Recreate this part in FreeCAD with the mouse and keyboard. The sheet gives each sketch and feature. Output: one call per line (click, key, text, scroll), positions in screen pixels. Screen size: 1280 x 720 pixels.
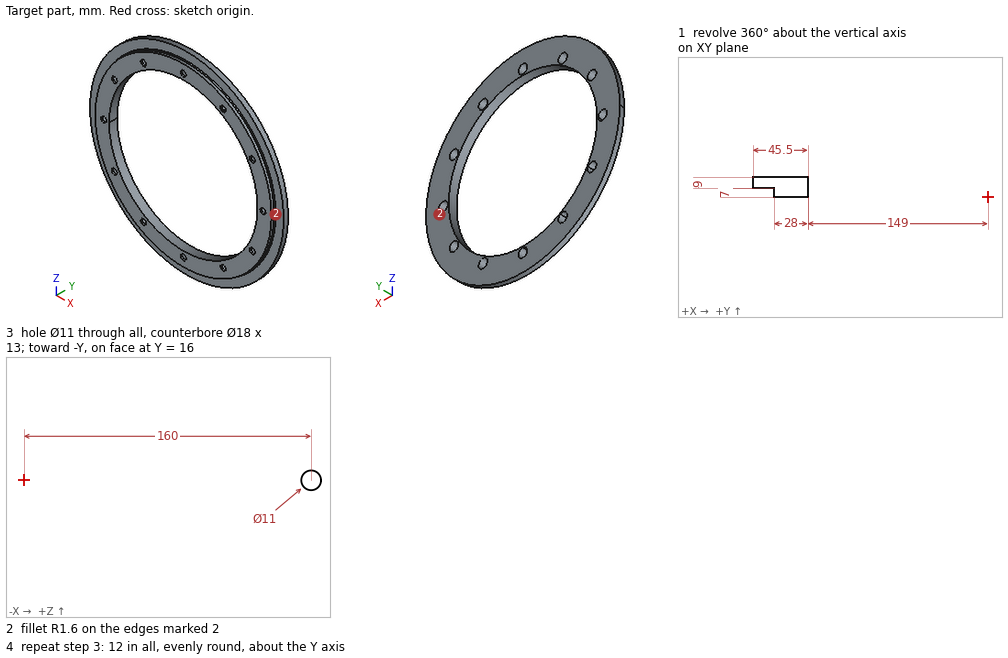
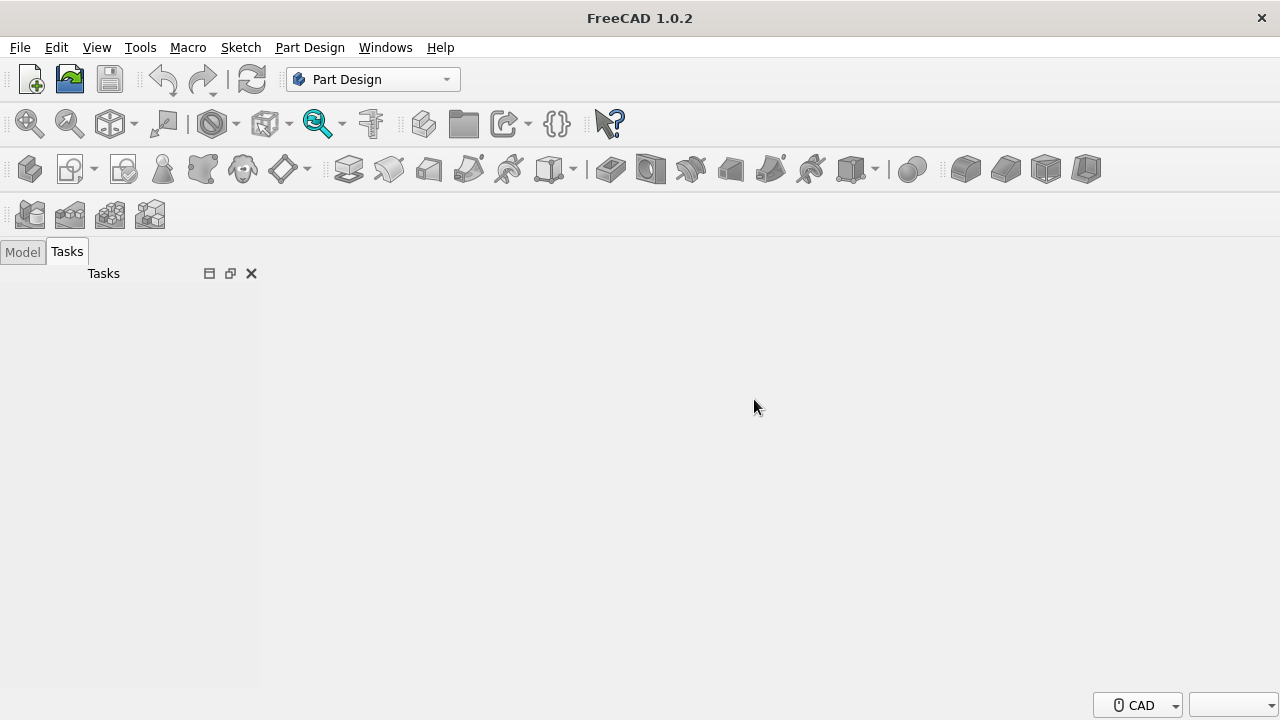
click(30, 80)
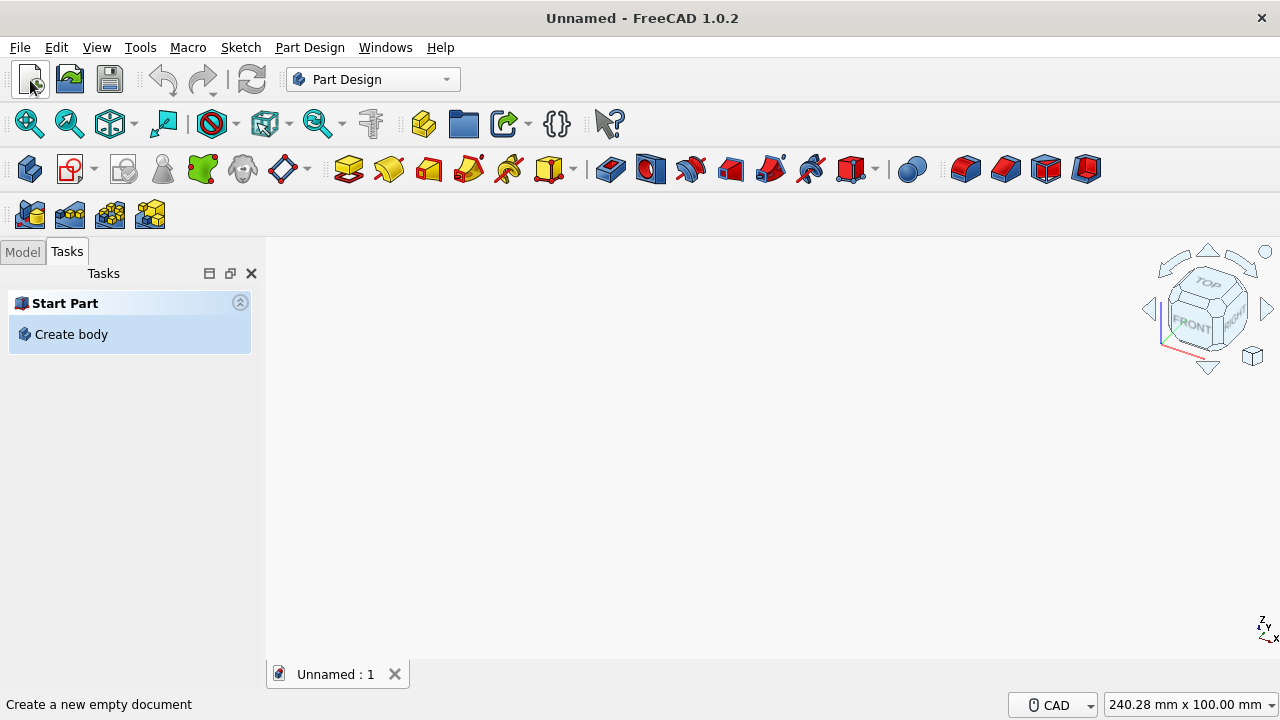
click(70, 170)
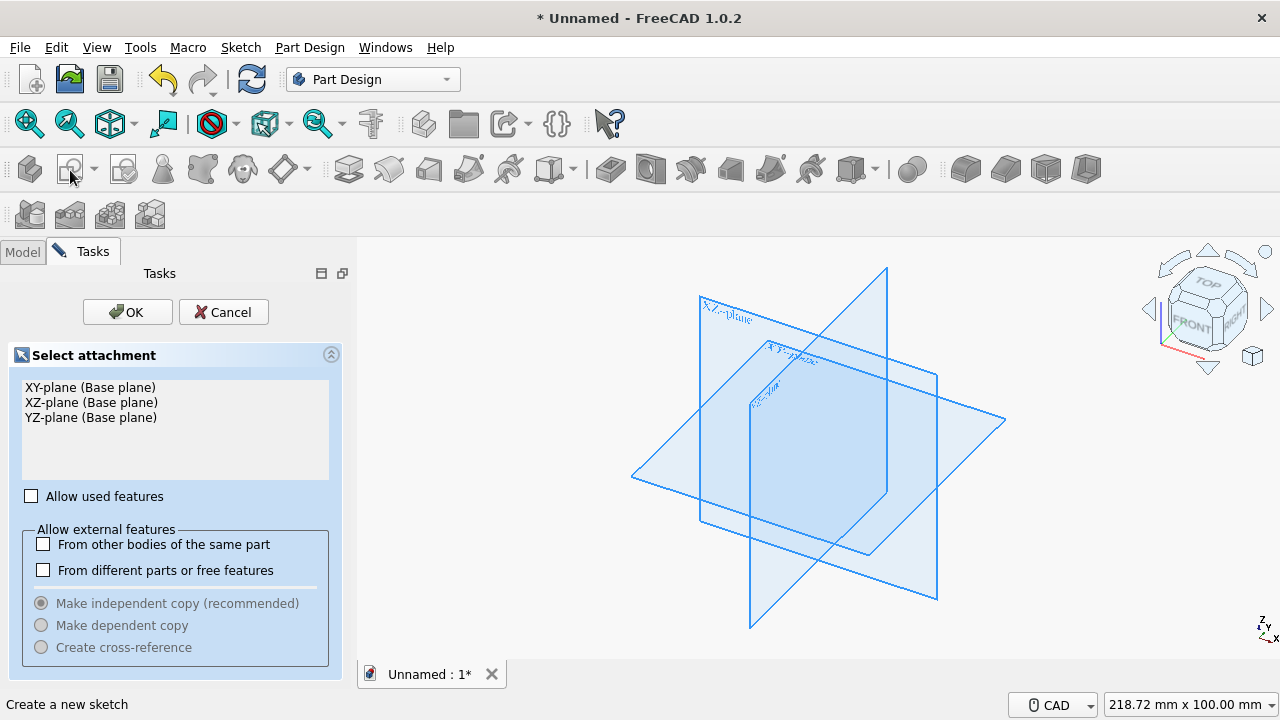
click(82, 388)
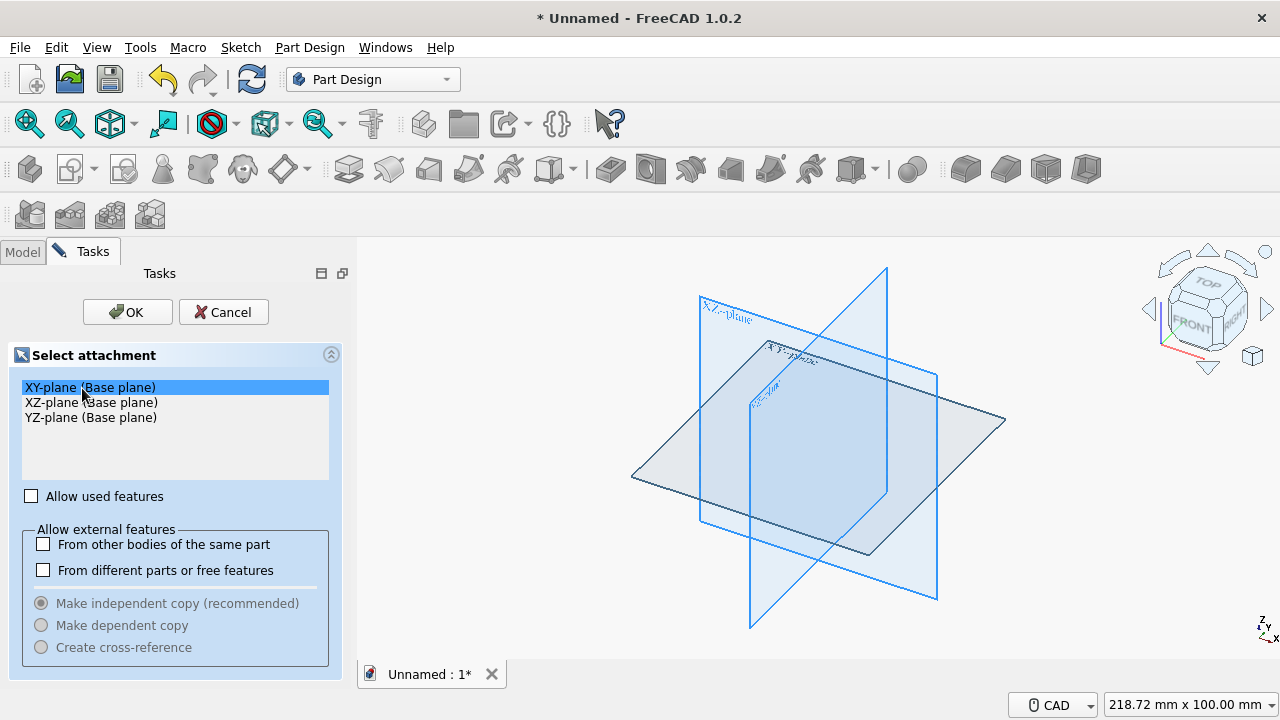
click(128, 312)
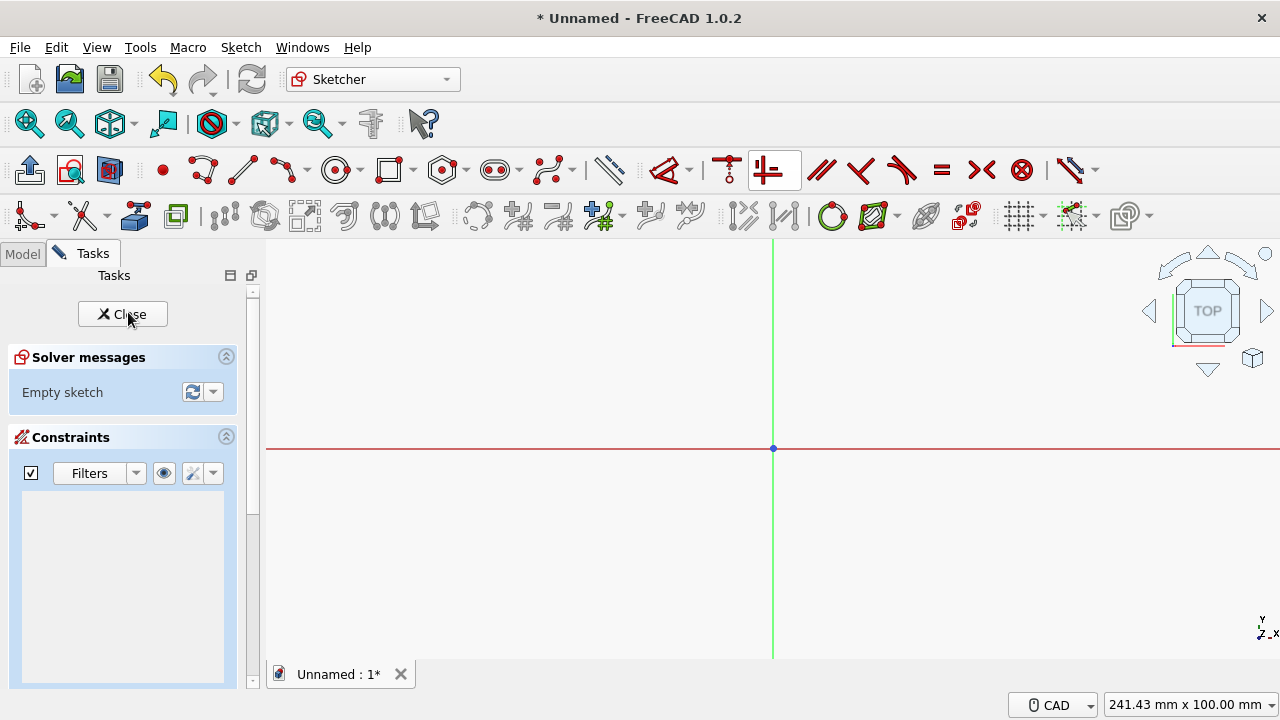
scroll(704, 449, down, 5)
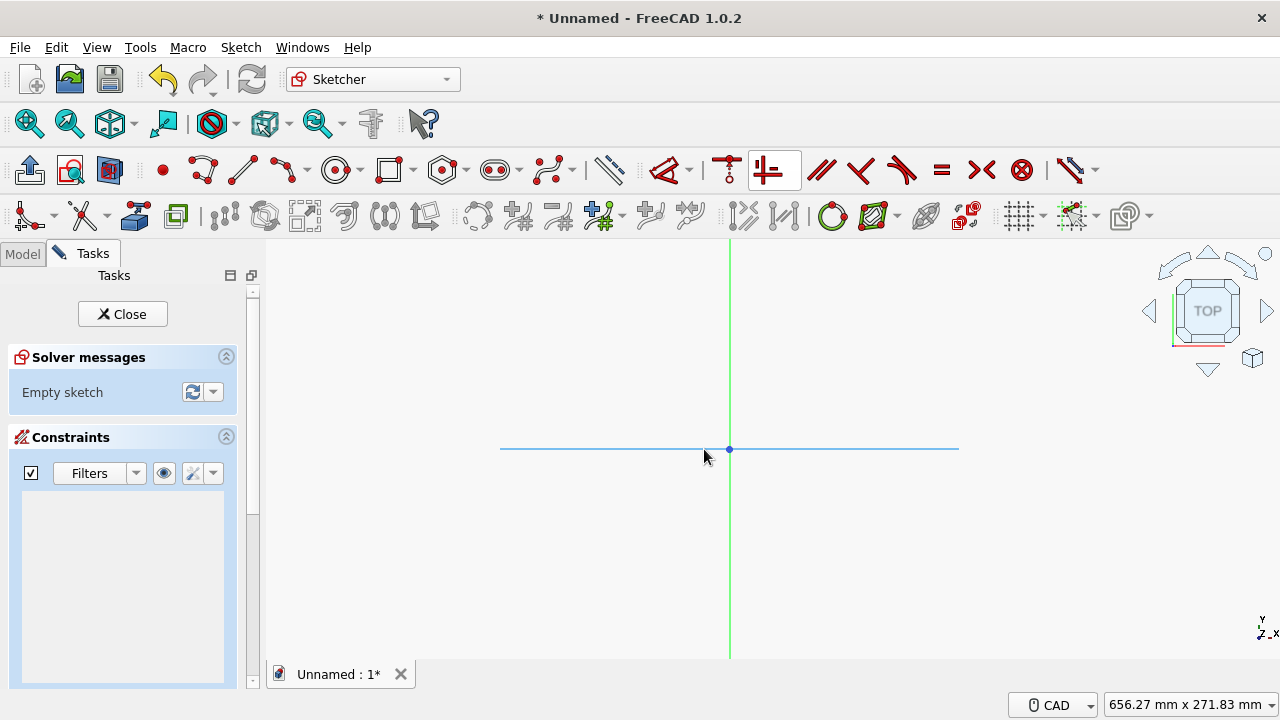
scroll(434, 435, up, 11)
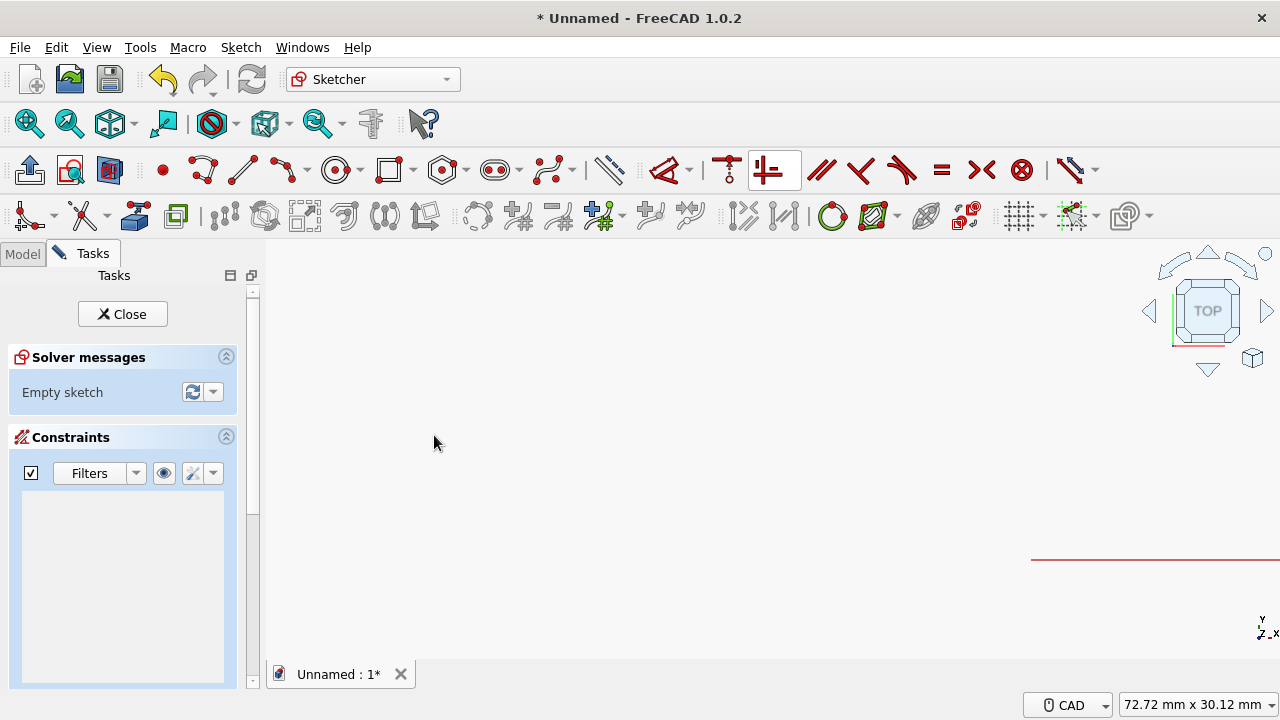
click(204, 170)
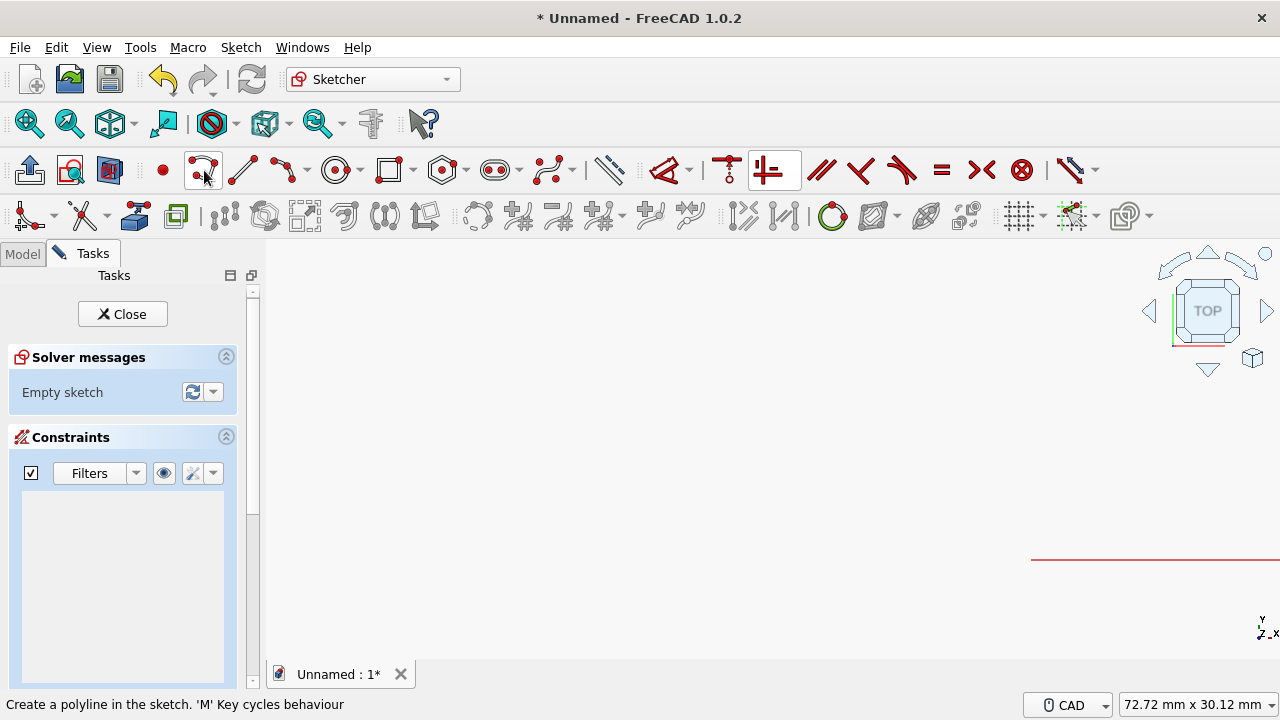
click(1023, 560)
click(1023, 337)
click(389, 337)
click(389, 463)
click(633, 463)
click(633, 551)
click(1023, 561)
key(Escape)
key(Escape)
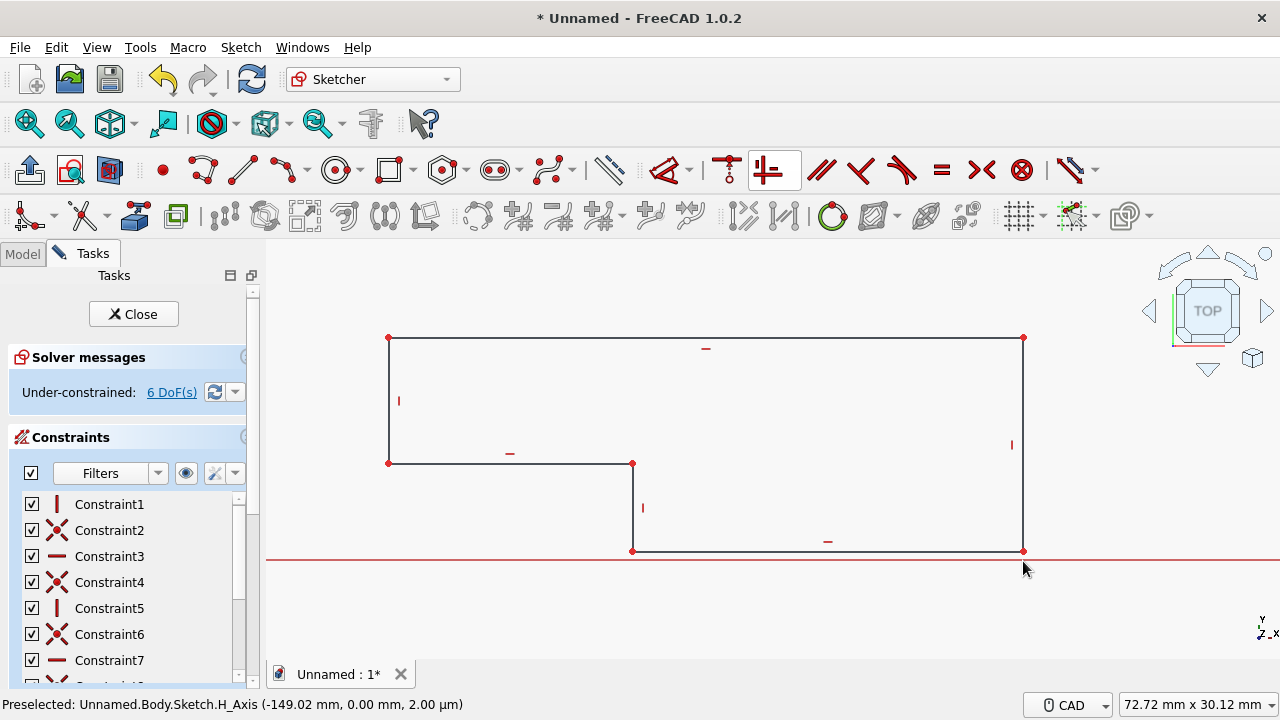
click(1023, 552)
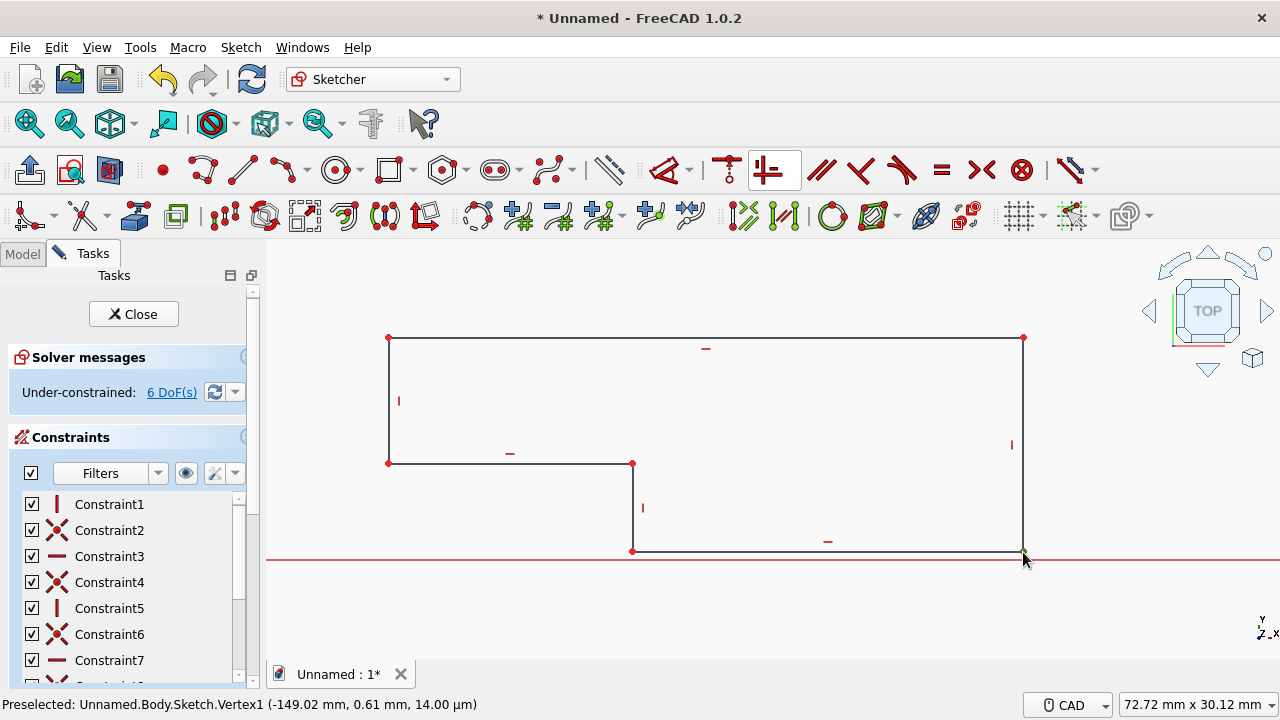
click(353, 560)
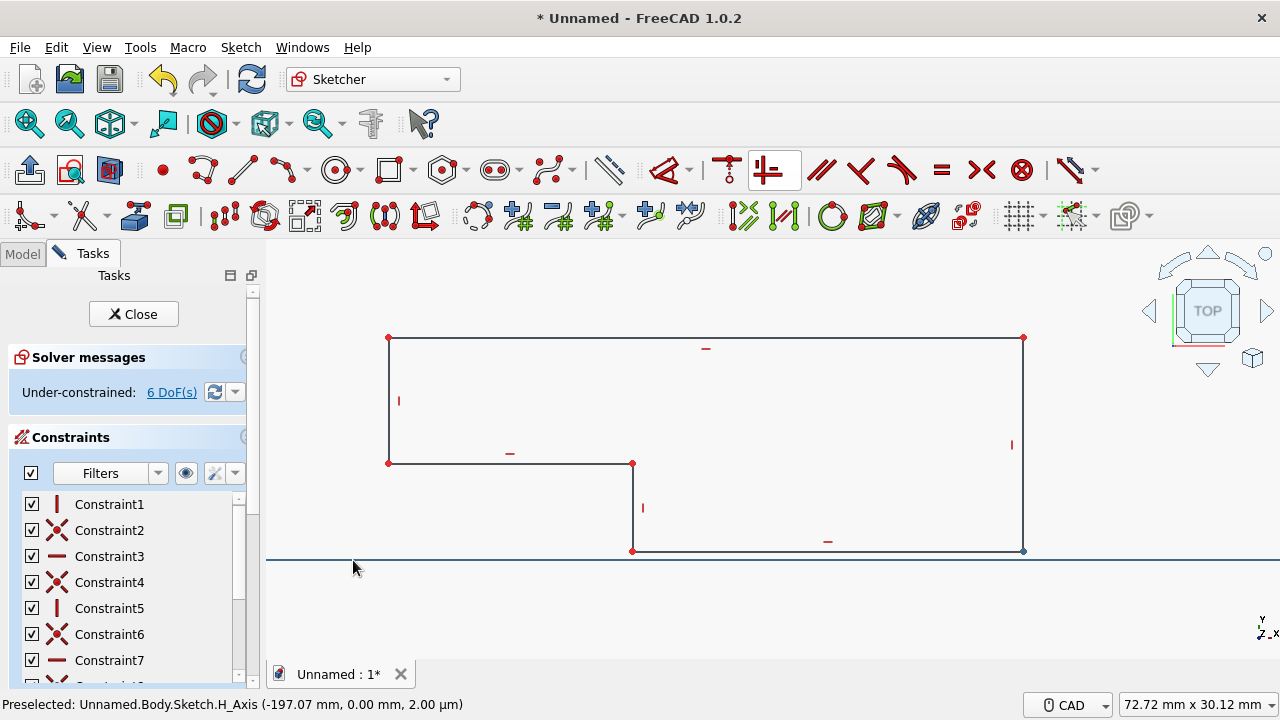
click(728, 170)